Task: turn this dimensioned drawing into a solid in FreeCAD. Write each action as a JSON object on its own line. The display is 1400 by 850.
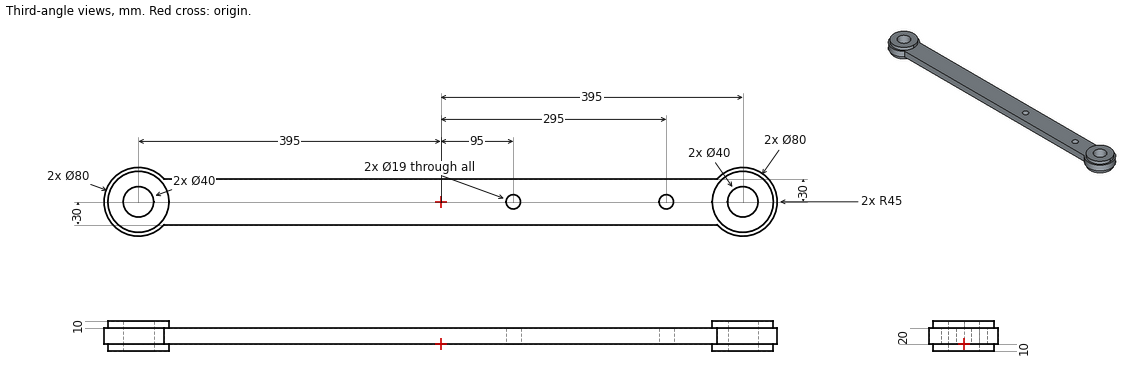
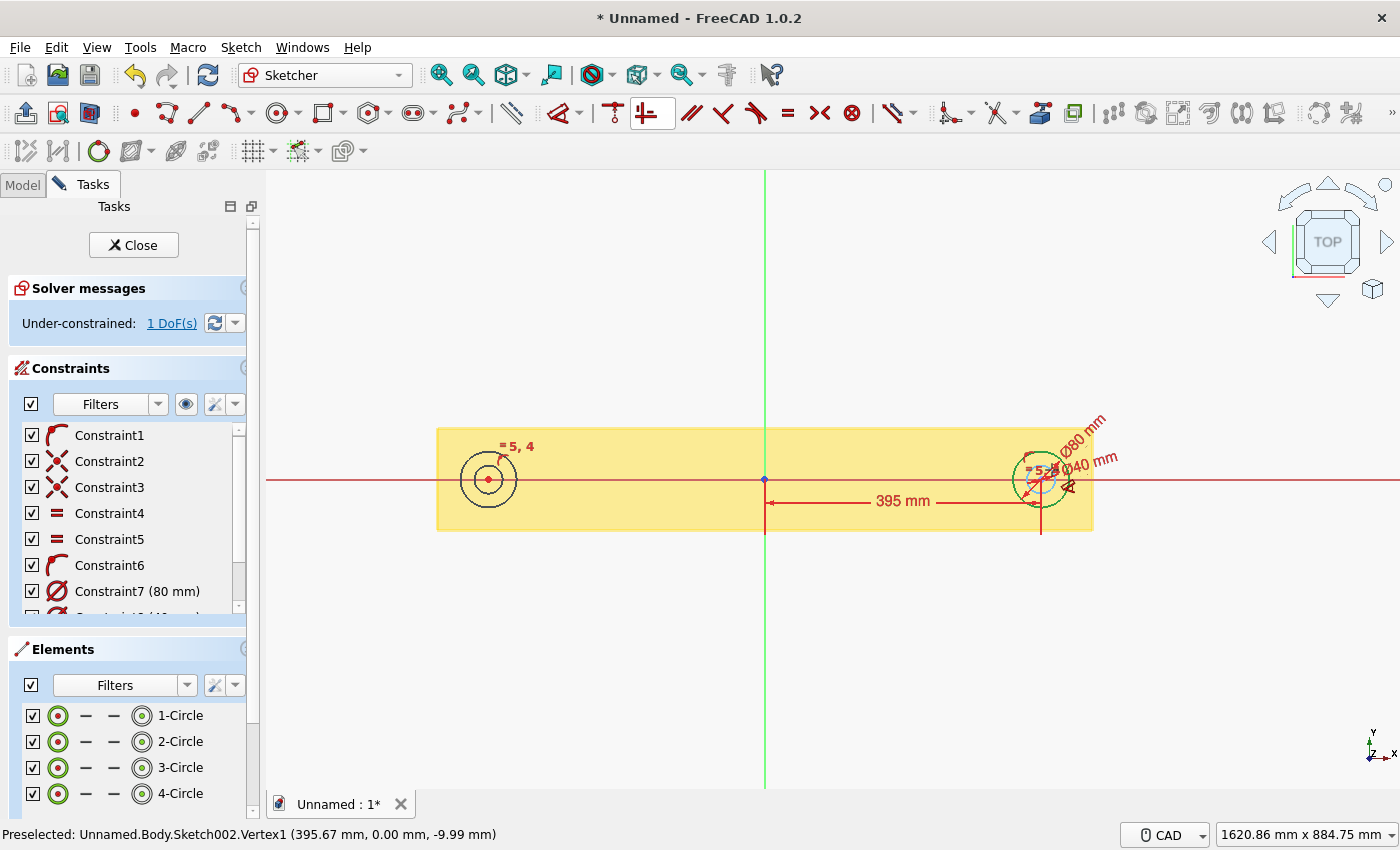
{"action": "left_click", "coordinate": [489, 480]}
{"action": "left_click", "coordinate": [627, 514]}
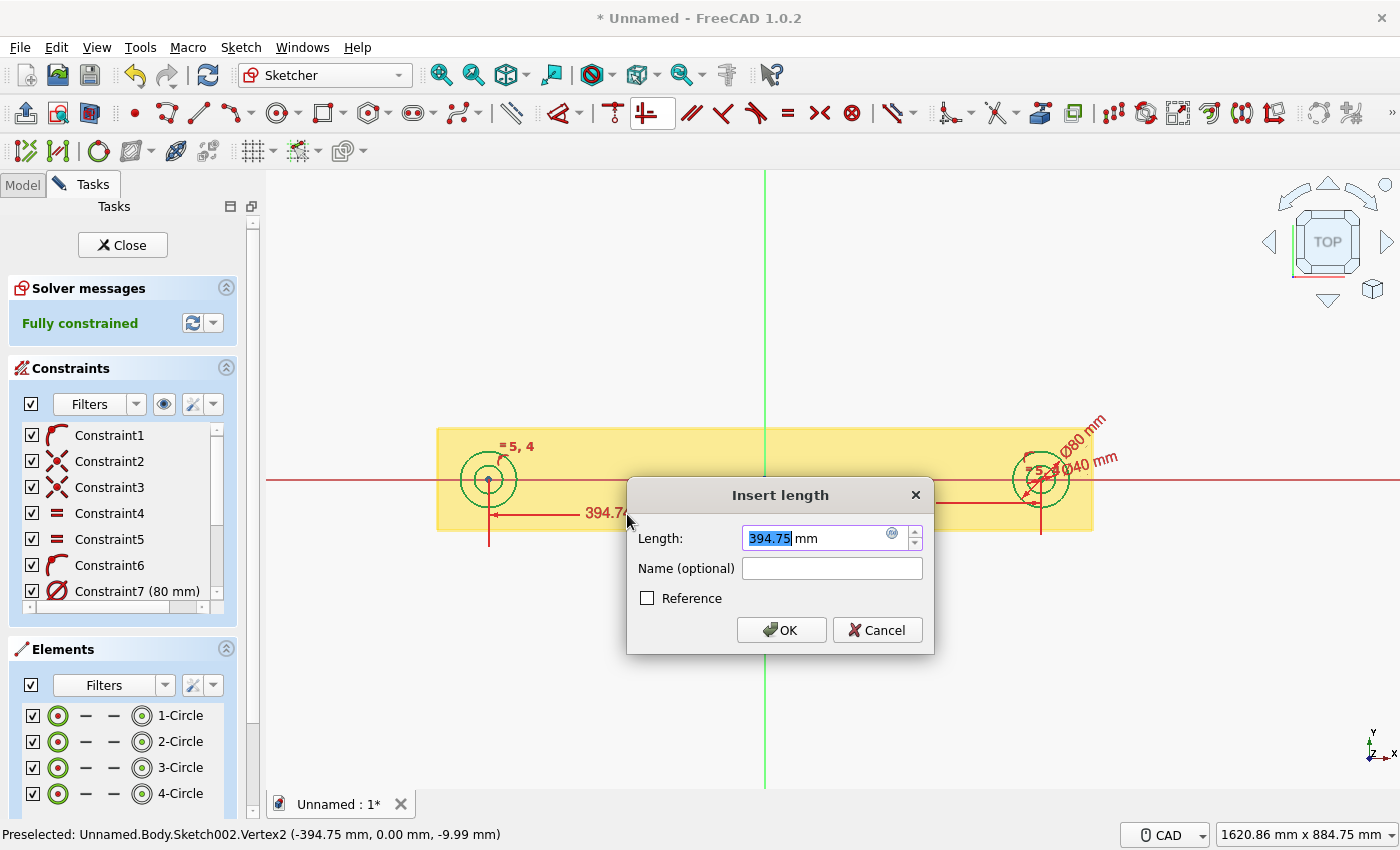
{"action": "type", "text": "395"}
{"action": "key", "text": "Return"}
{"action": "key", "text": "Escape"}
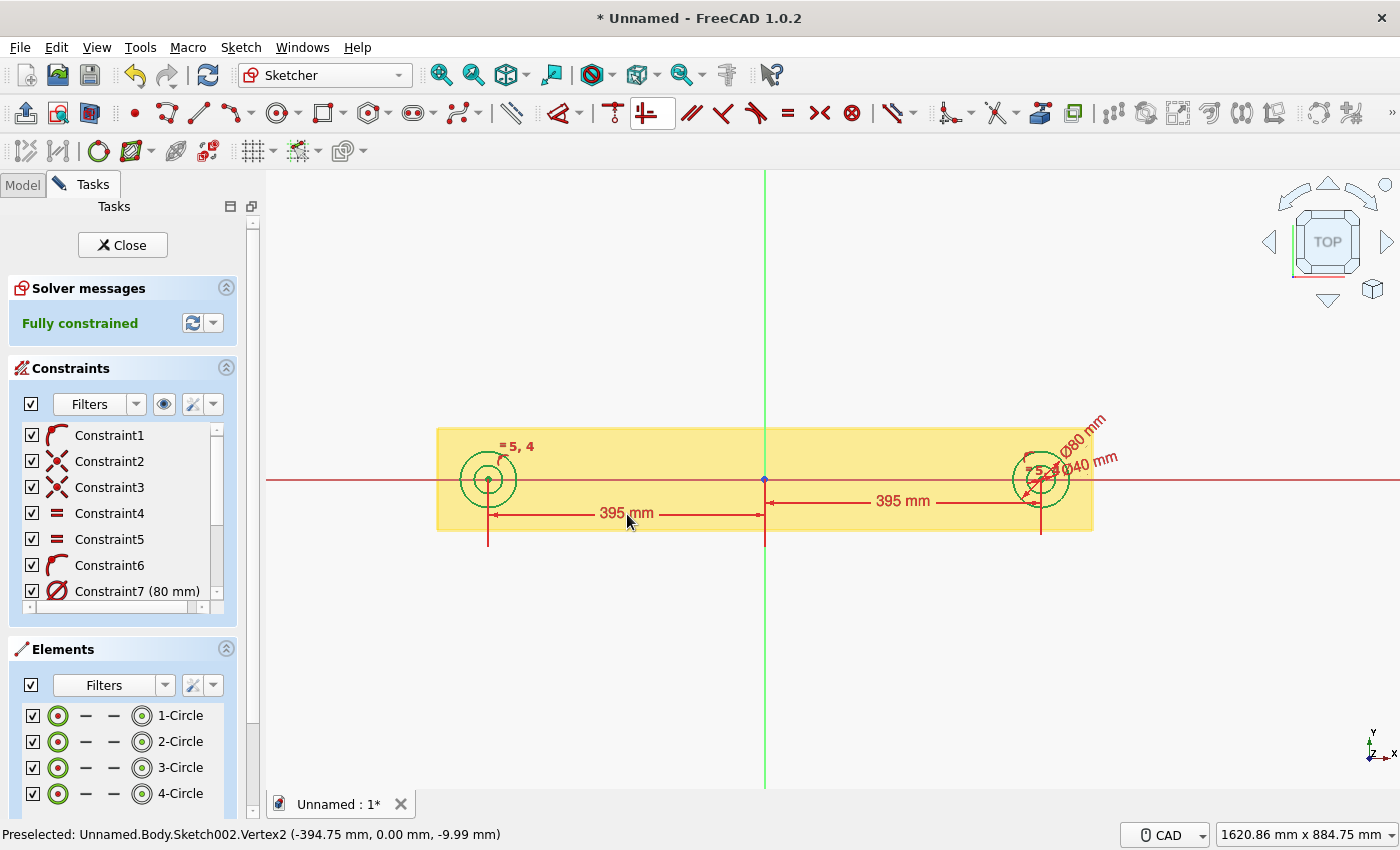
{"action": "left_click", "coordinate": [123, 245]}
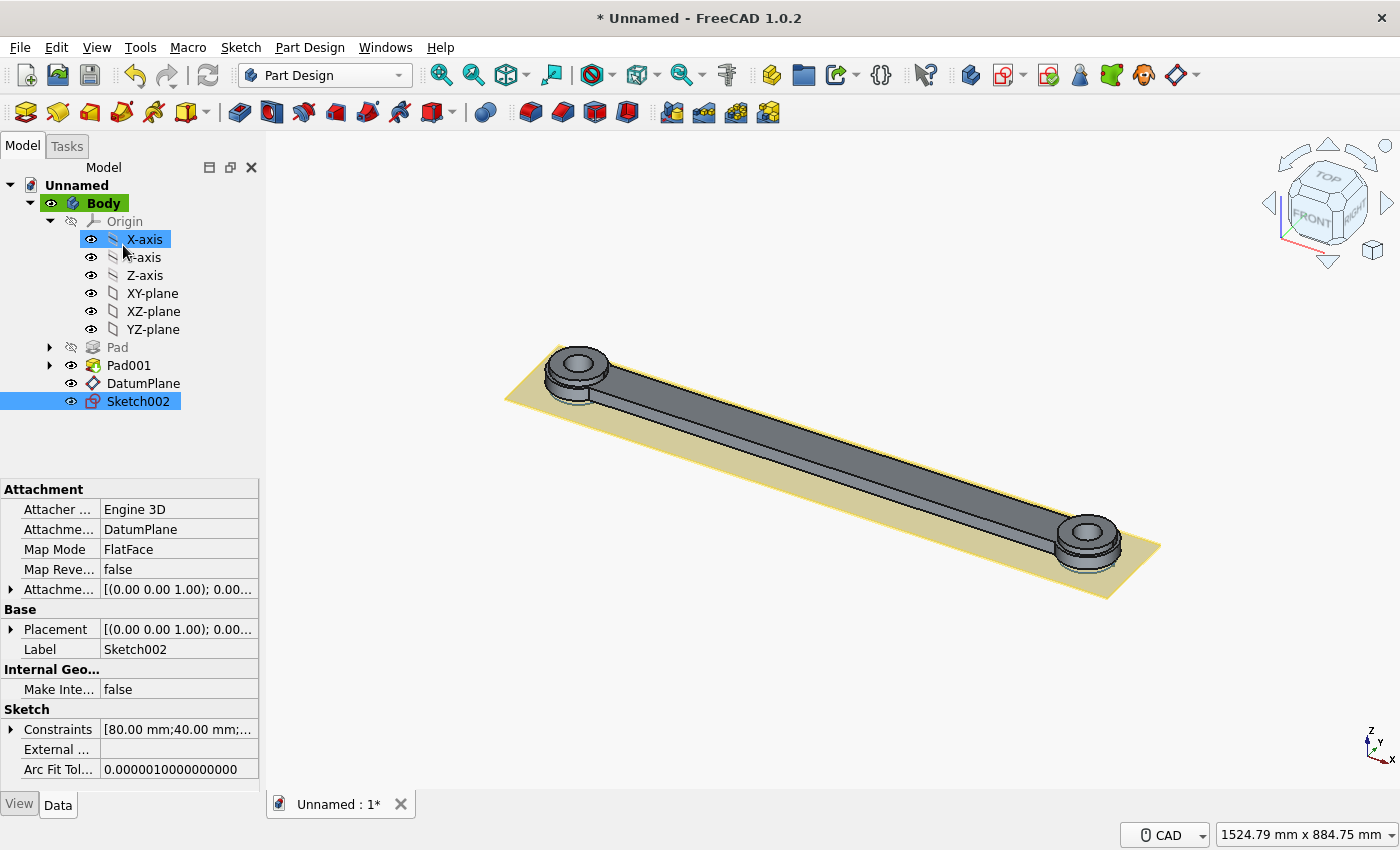
{"action": "left_click", "coordinate": [26, 112]}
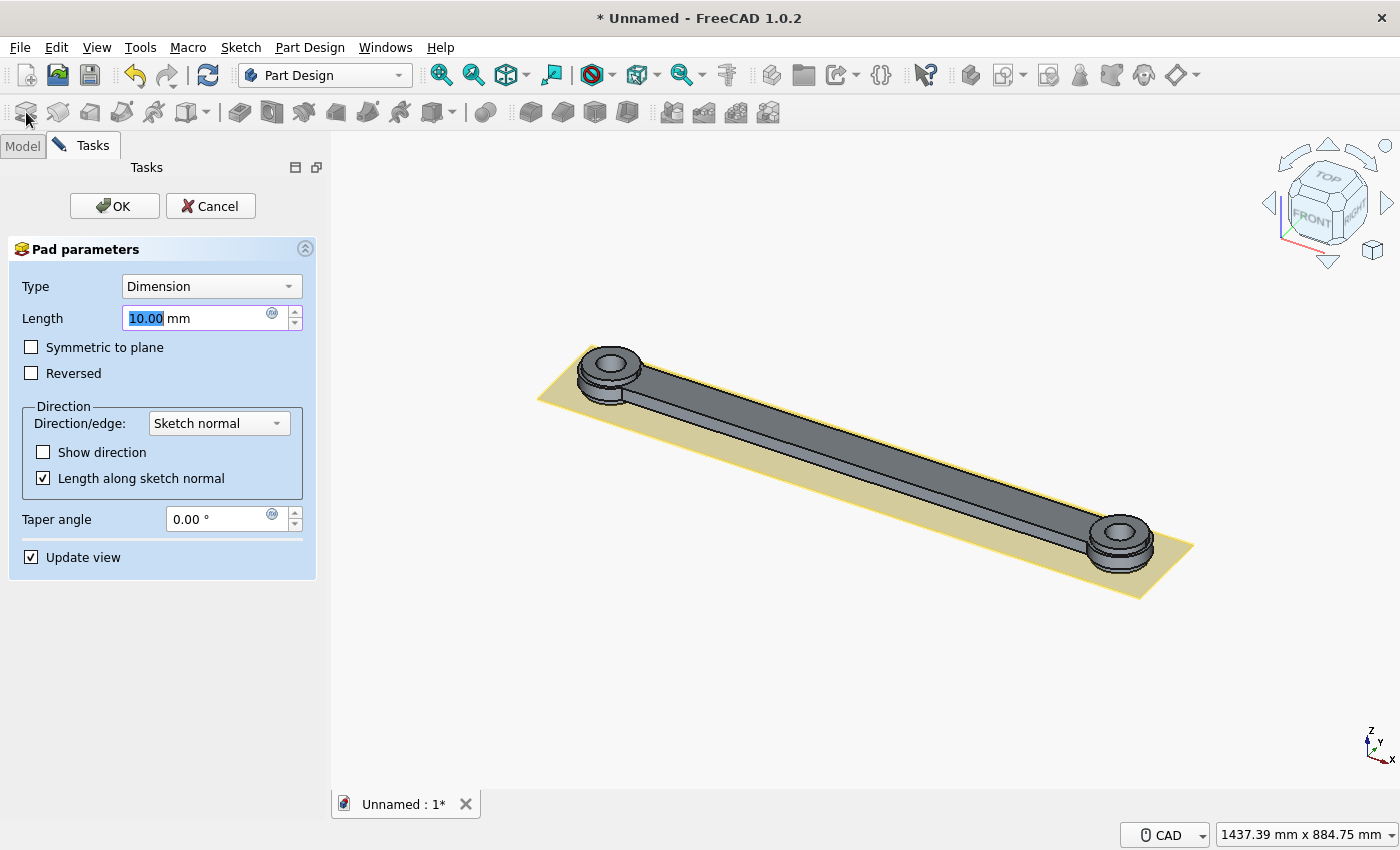
{"action": "type", "text": "10"}
{"action": "key", "text": "Tab"}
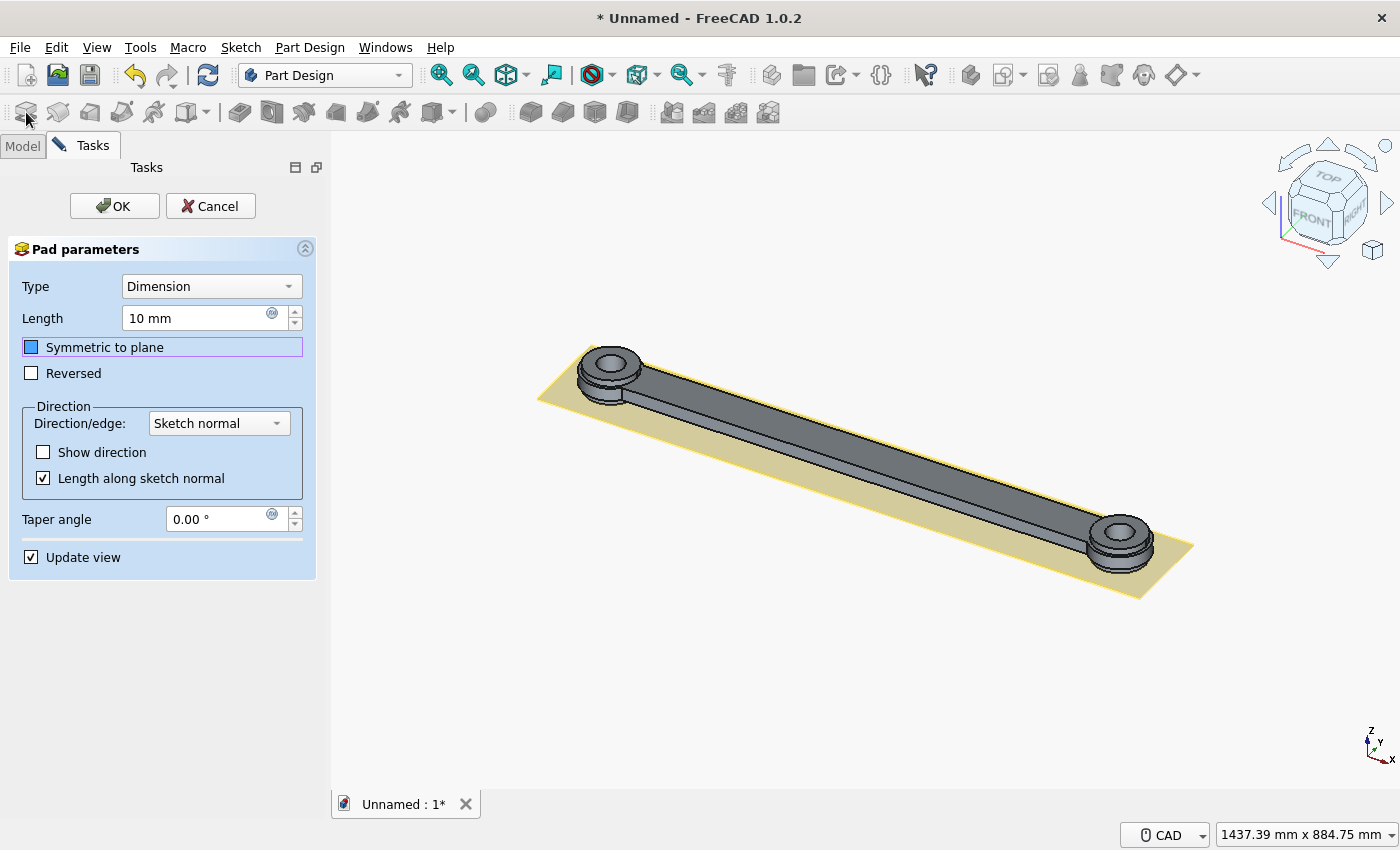
{"action": "left_click", "coordinate": [115, 206]}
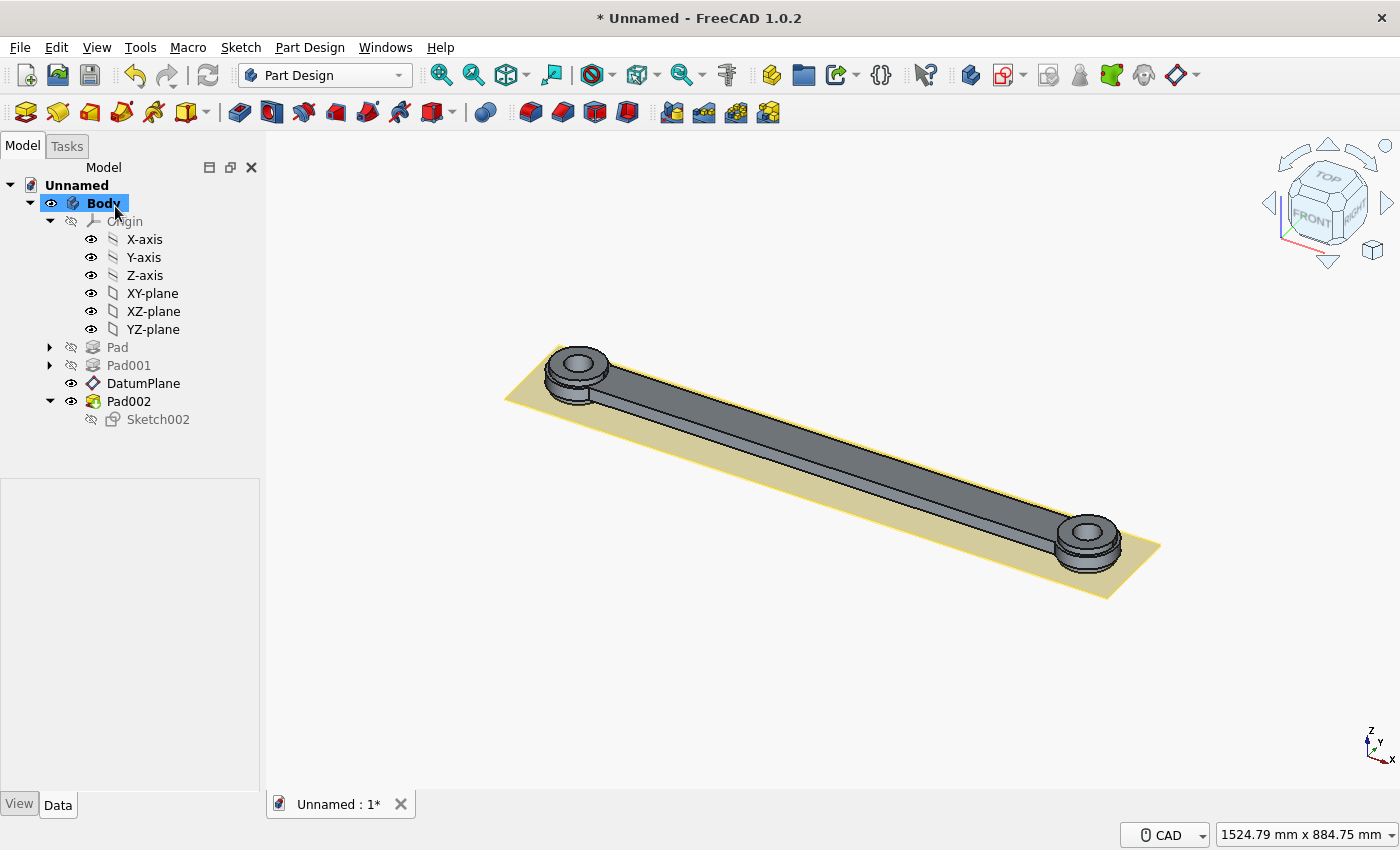
{"action": "left_click", "coordinate": [116, 383]}
{"action": "key", "text": "space"}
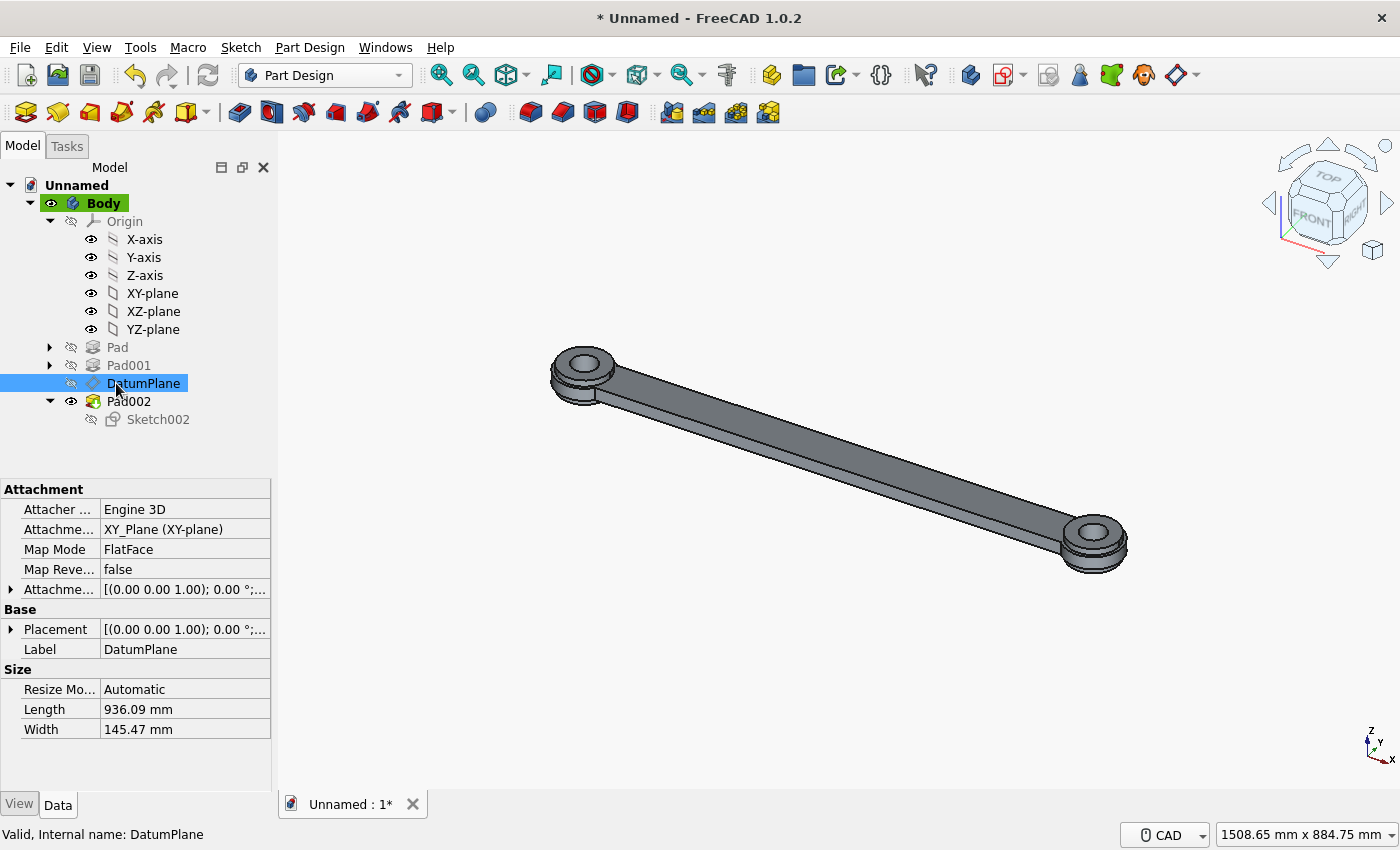
{"action": "left_click", "coordinate": [1001, 507]}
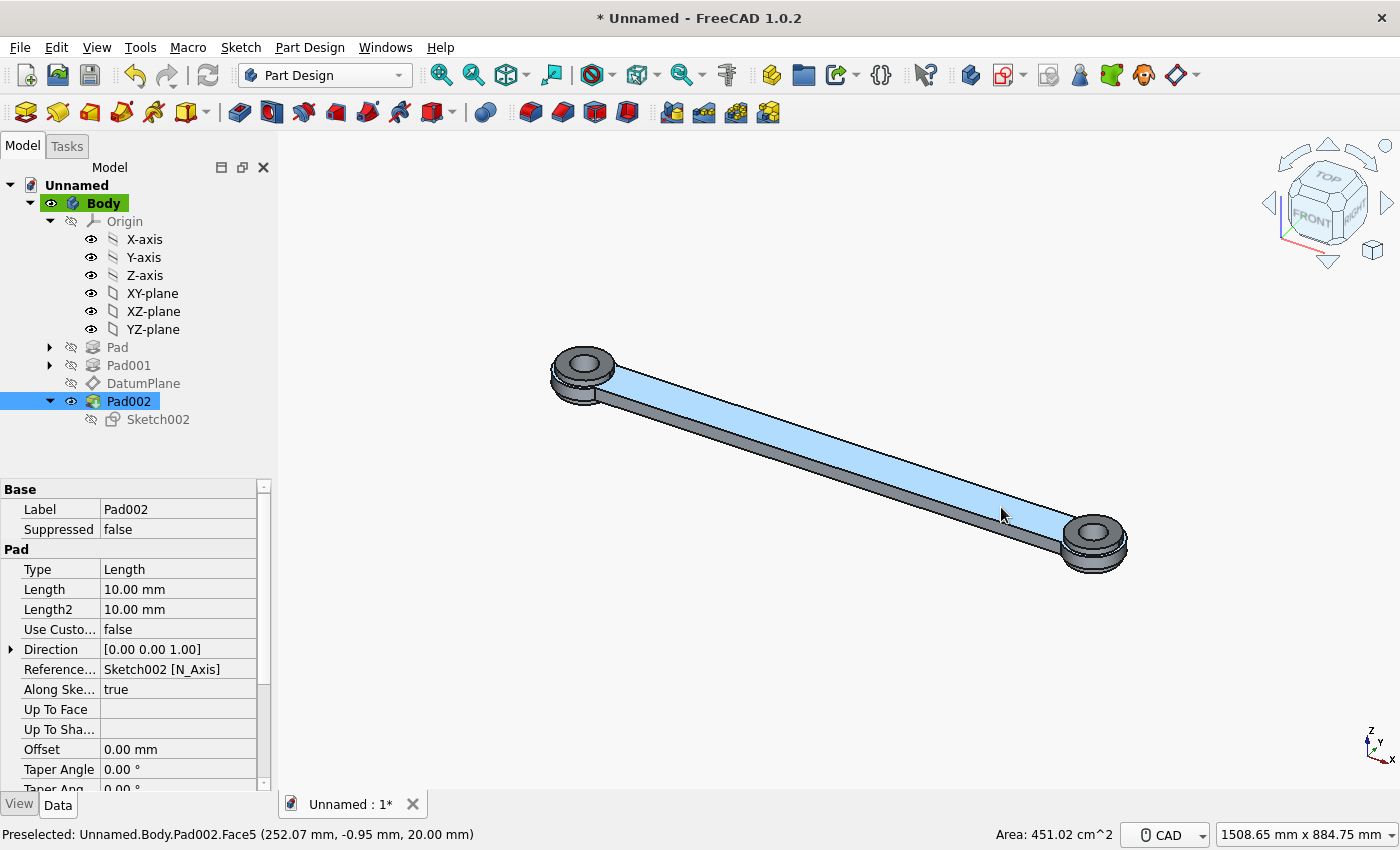
{"action": "left_click", "coordinate": [1004, 76]}